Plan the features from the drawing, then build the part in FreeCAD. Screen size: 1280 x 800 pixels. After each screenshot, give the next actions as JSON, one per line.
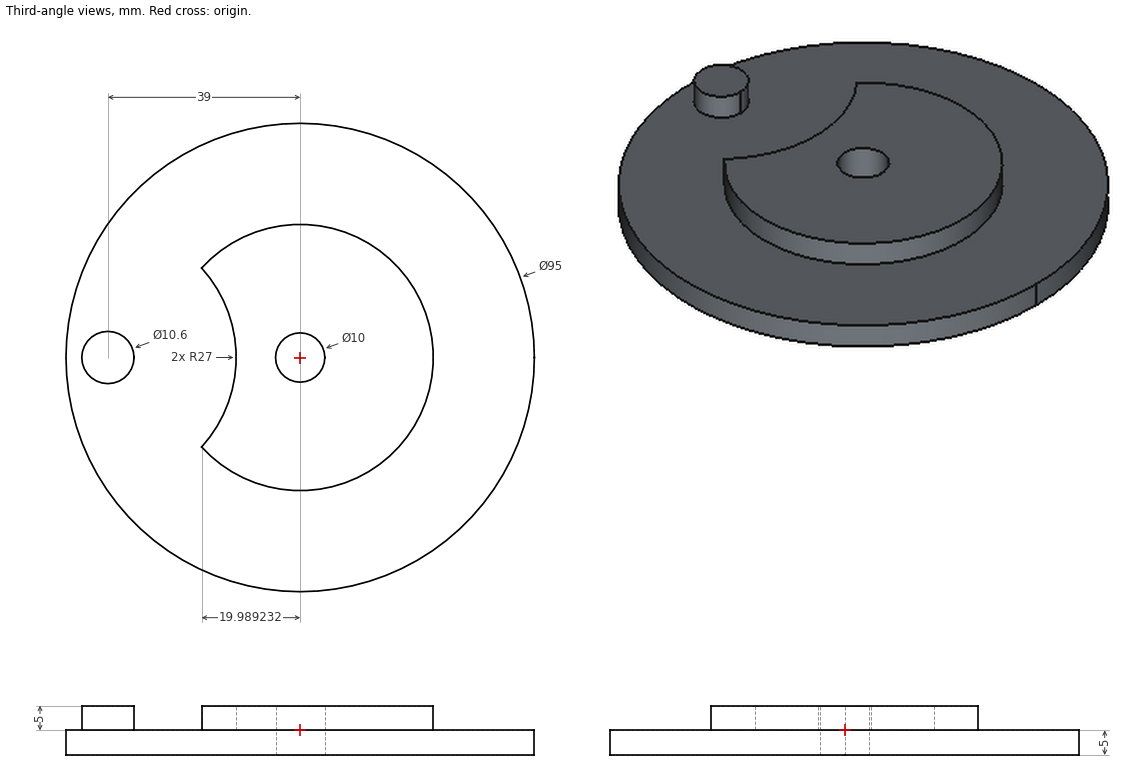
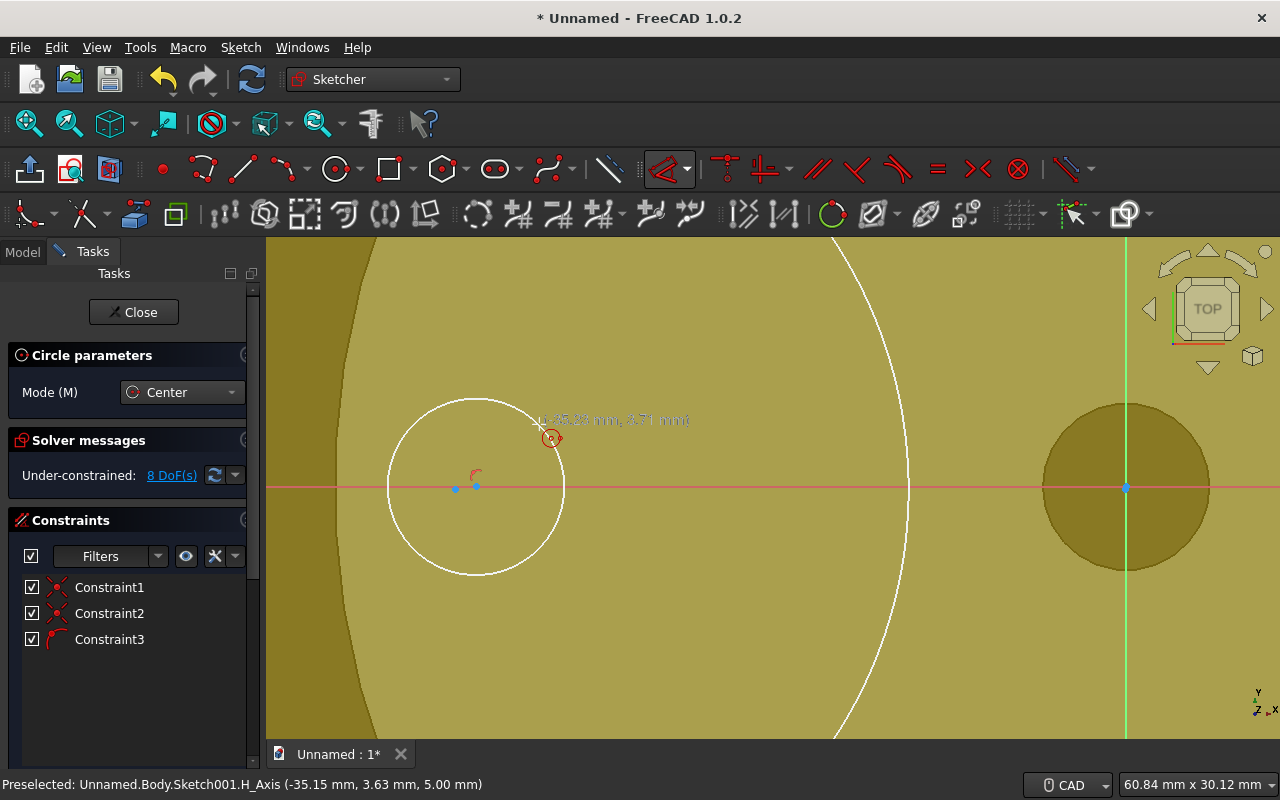
{"action": "scroll", "coordinate": [478, 489], "scroll_direction": "down", "scroll_amount": 4}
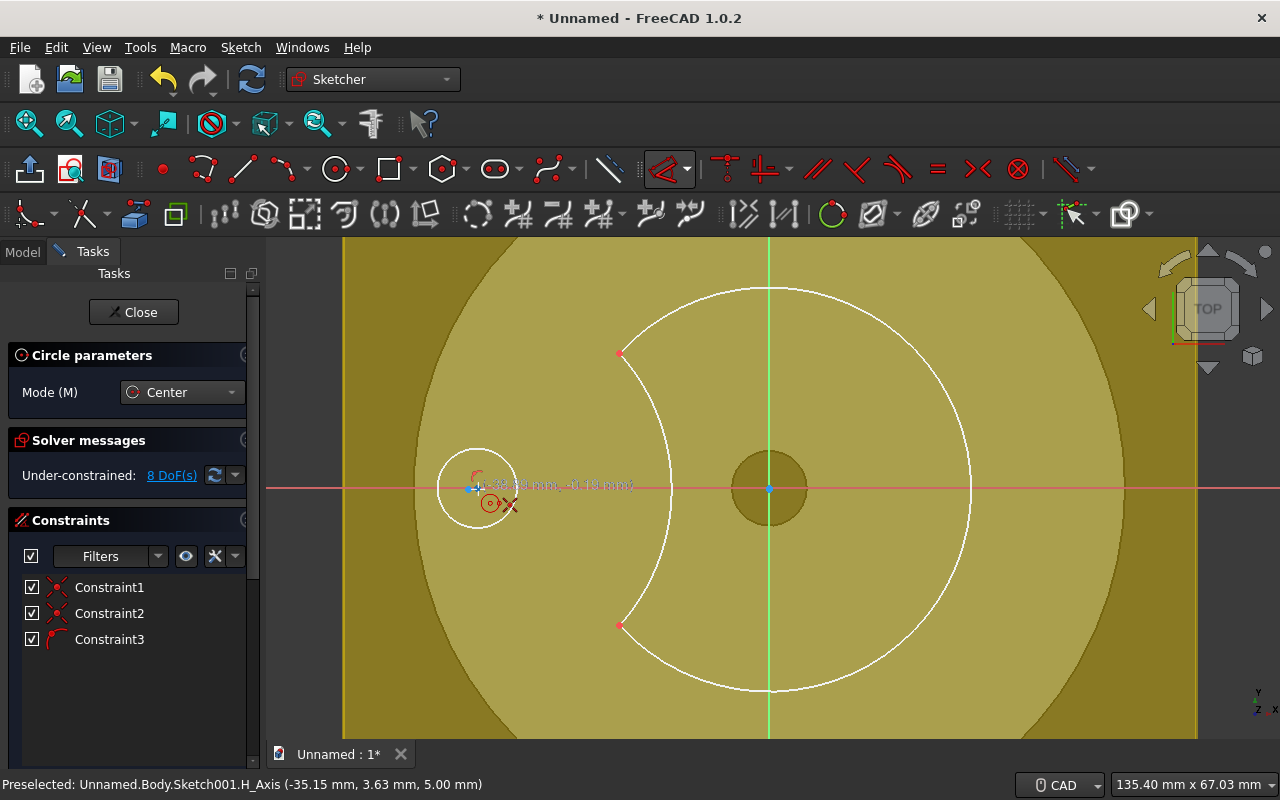
{"action": "left_click", "coordinate": [769, 488]}
{"action": "left_click", "coordinate": [796, 462]}
{"action": "key", "text": "Escape"}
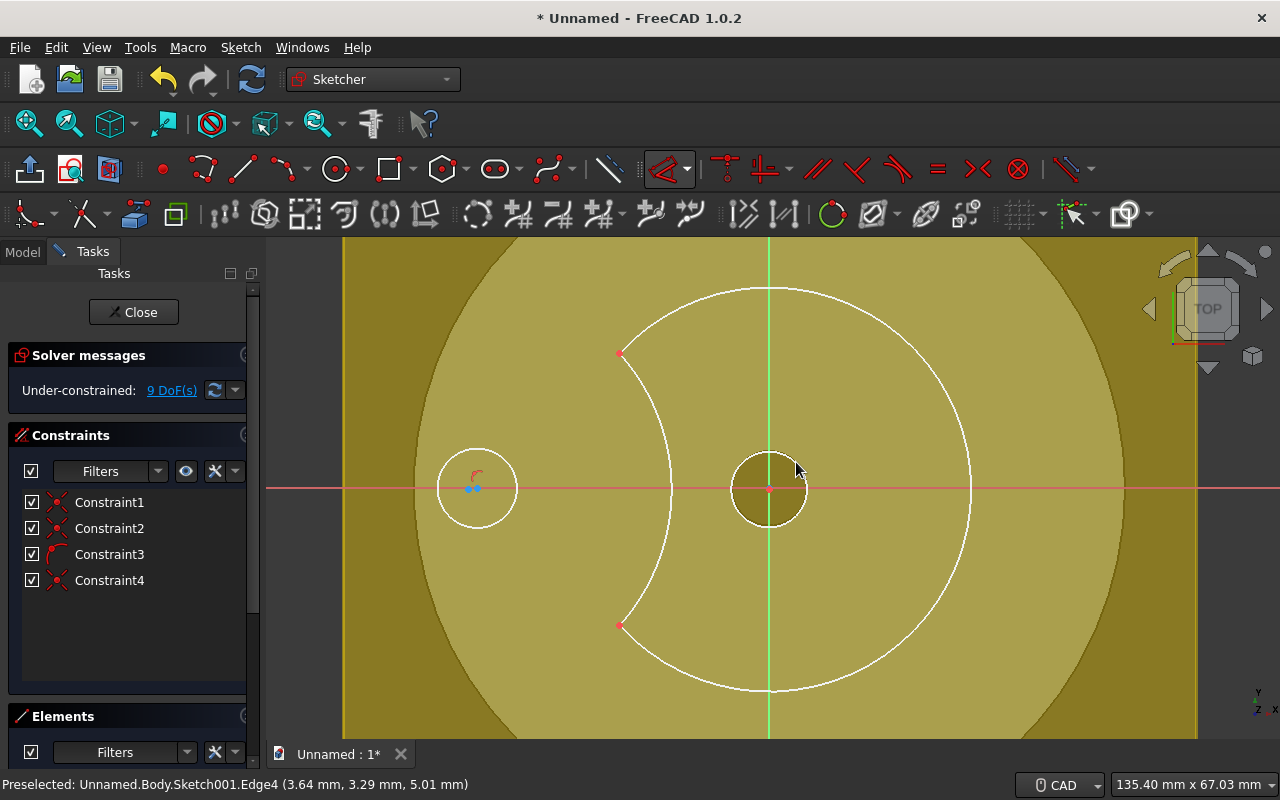
{"action": "left_click_drag", "start_coordinate": [759, 478], "coordinate": [779, 500]}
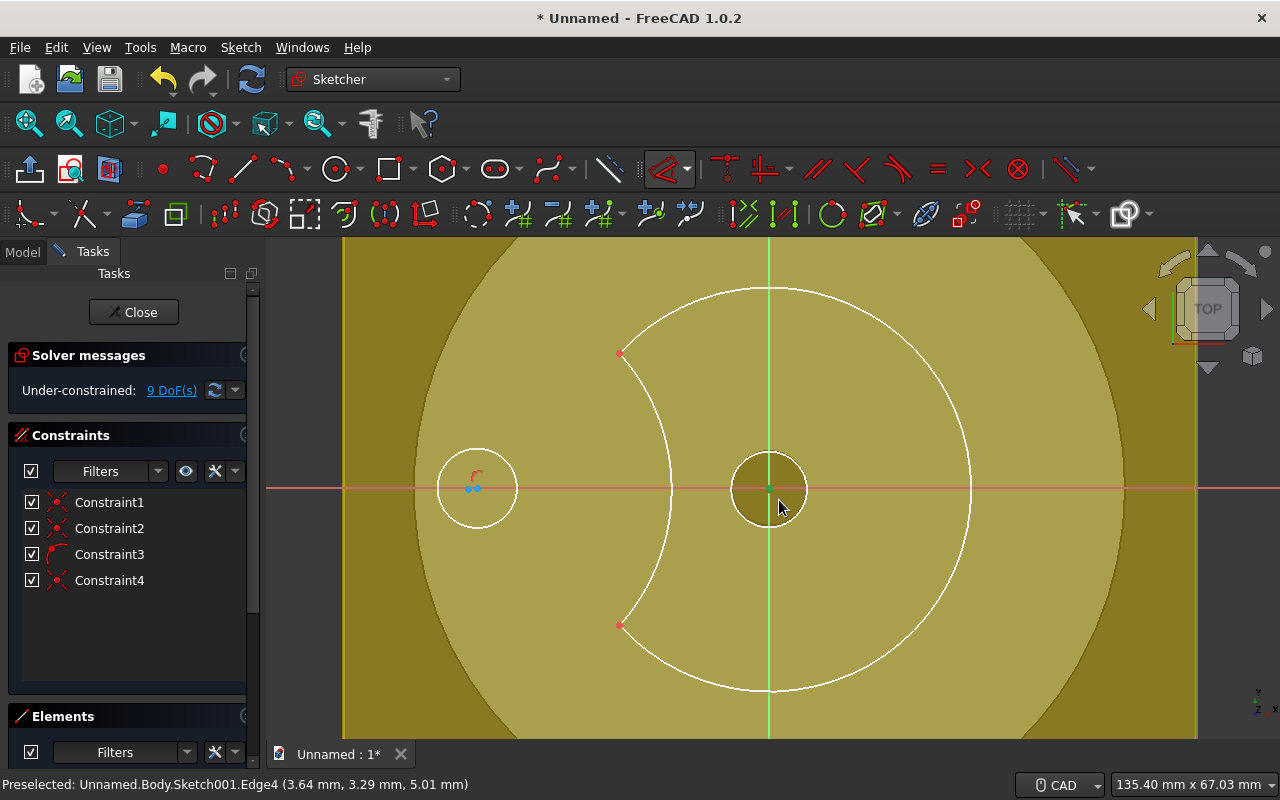
{"action": "key", "text": "c"}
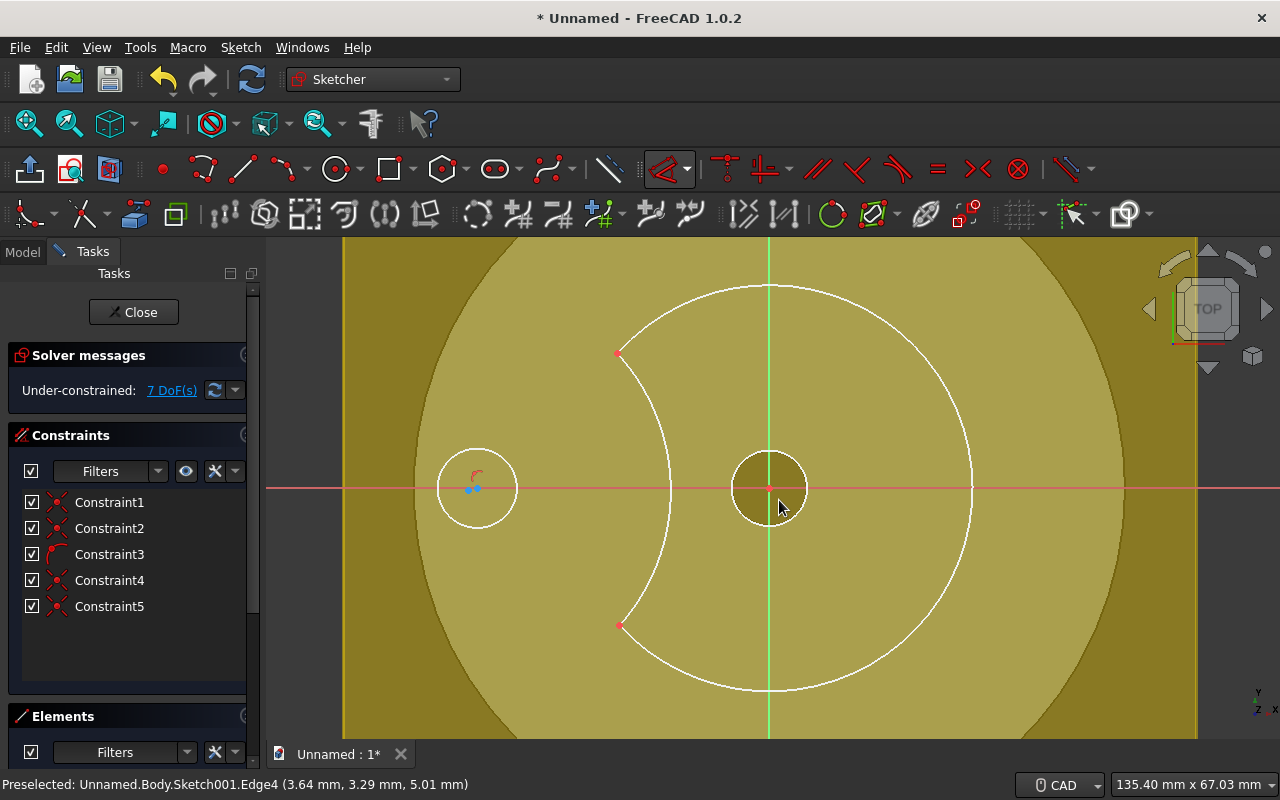
{"action": "left_click", "coordinate": [663, 548]}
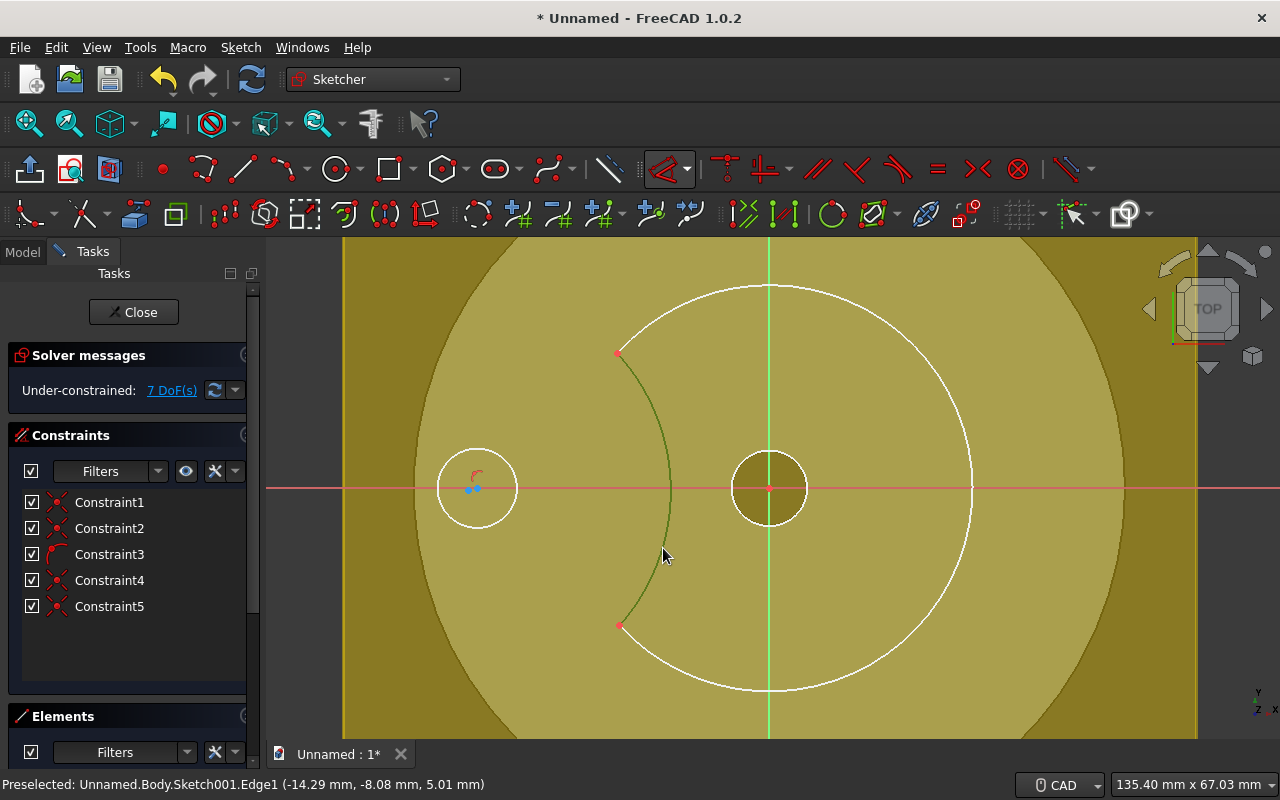
{"action": "left_click", "coordinate": [887, 654]}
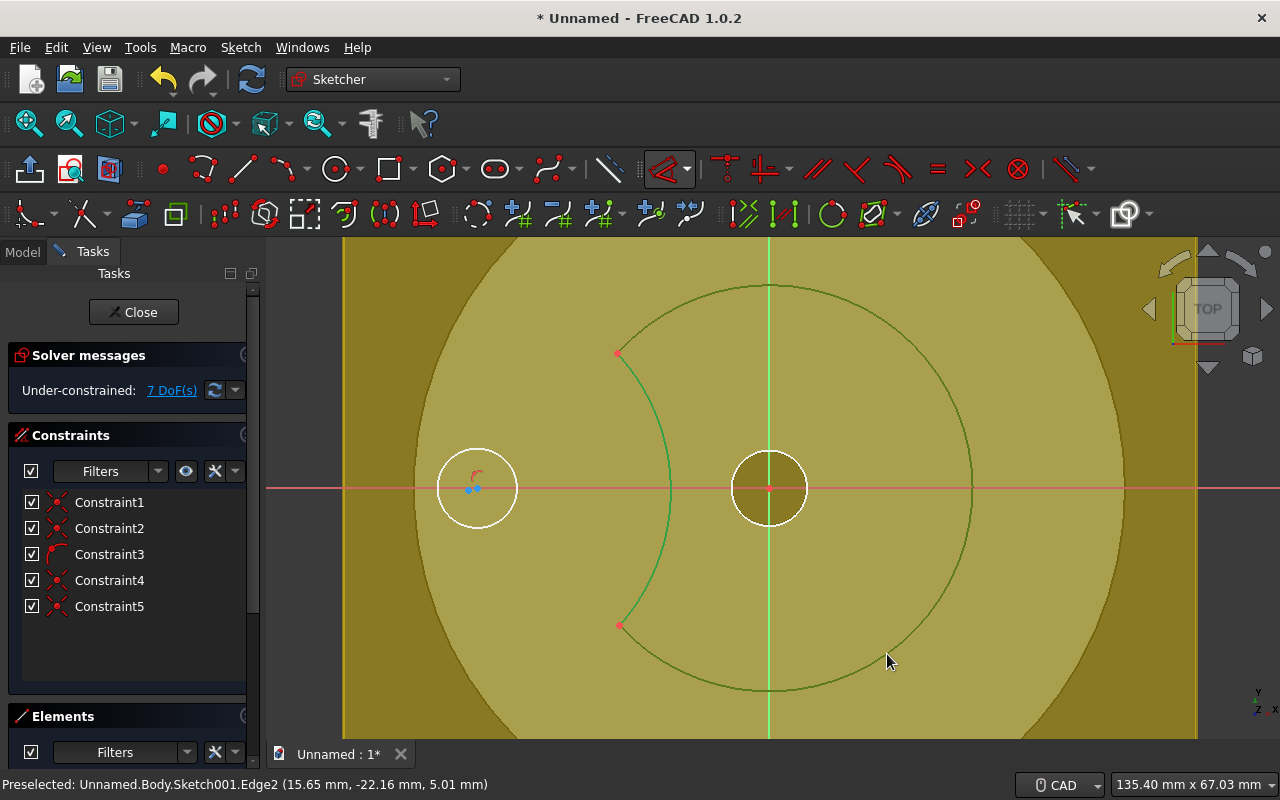
{"action": "key", "text": "e"}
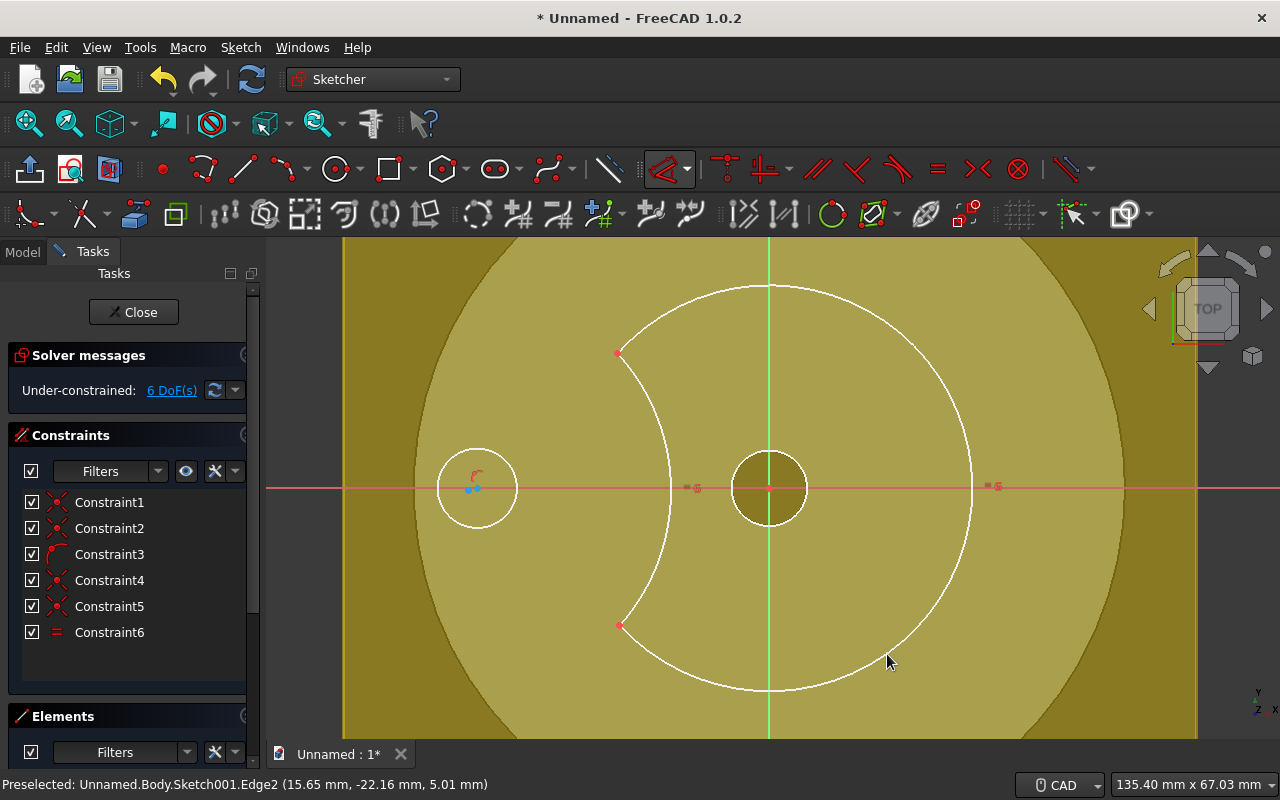
{"action": "scroll", "coordinate": [468, 491], "scroll_direction": "up", "scroll_amount": 2}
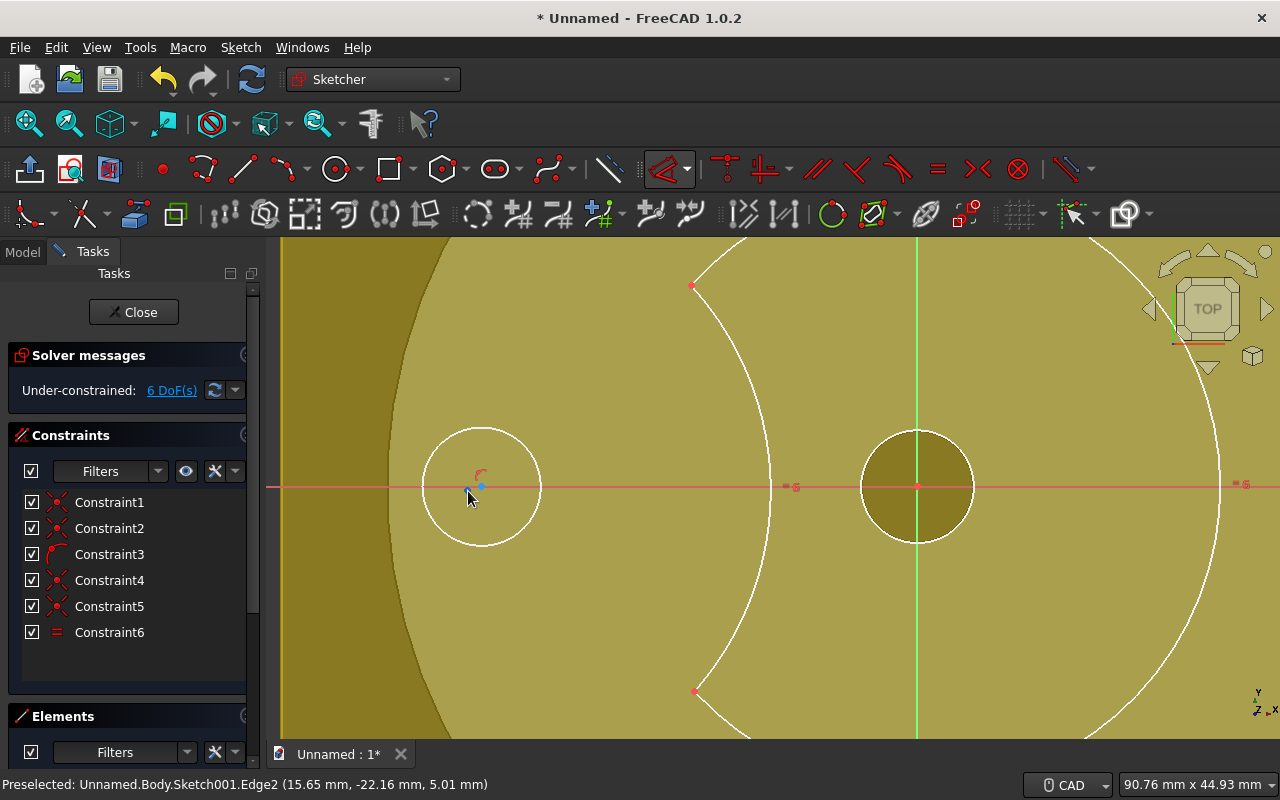
{"action": "left_click", "coordinate": [468, 490]}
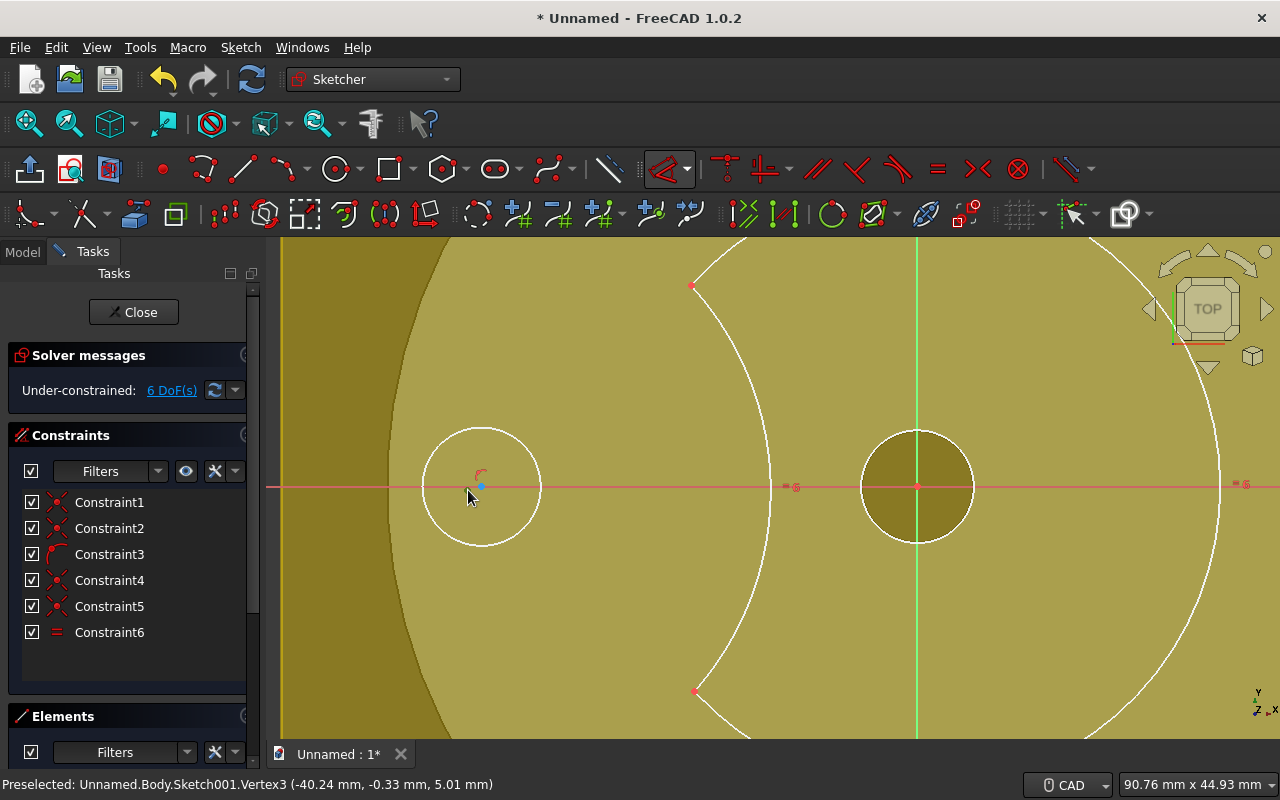
{"action": "left_click", "coordinate": [353, 487]}